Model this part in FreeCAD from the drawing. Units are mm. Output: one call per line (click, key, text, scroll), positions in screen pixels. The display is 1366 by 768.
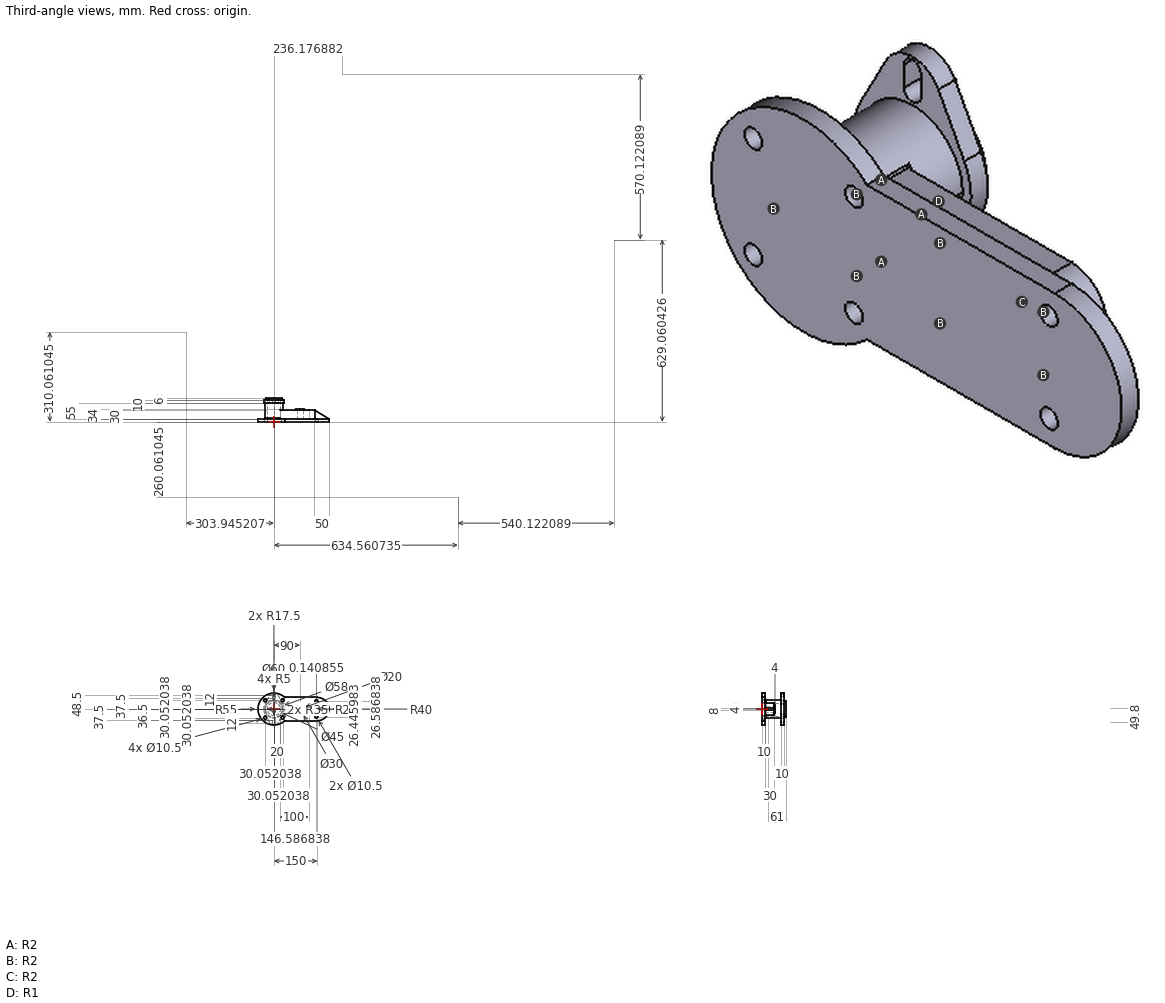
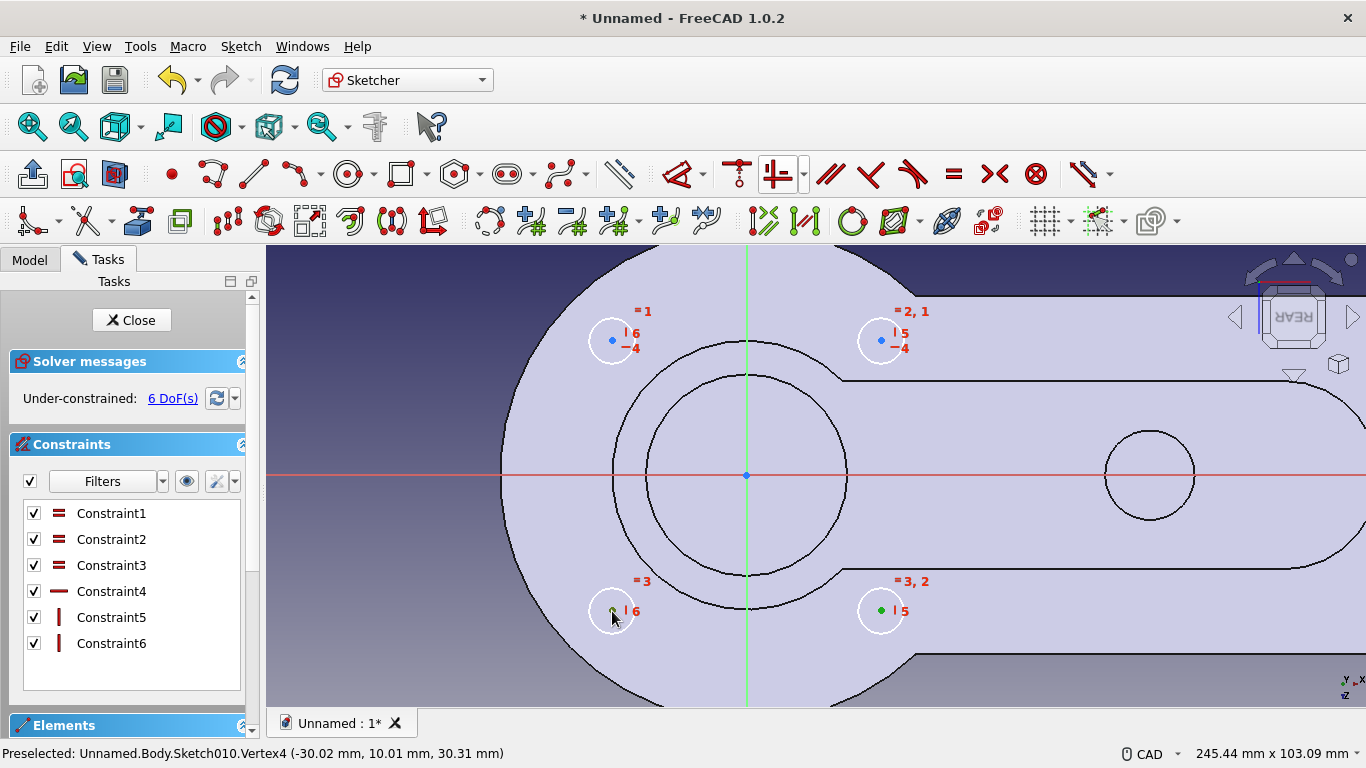
key(h)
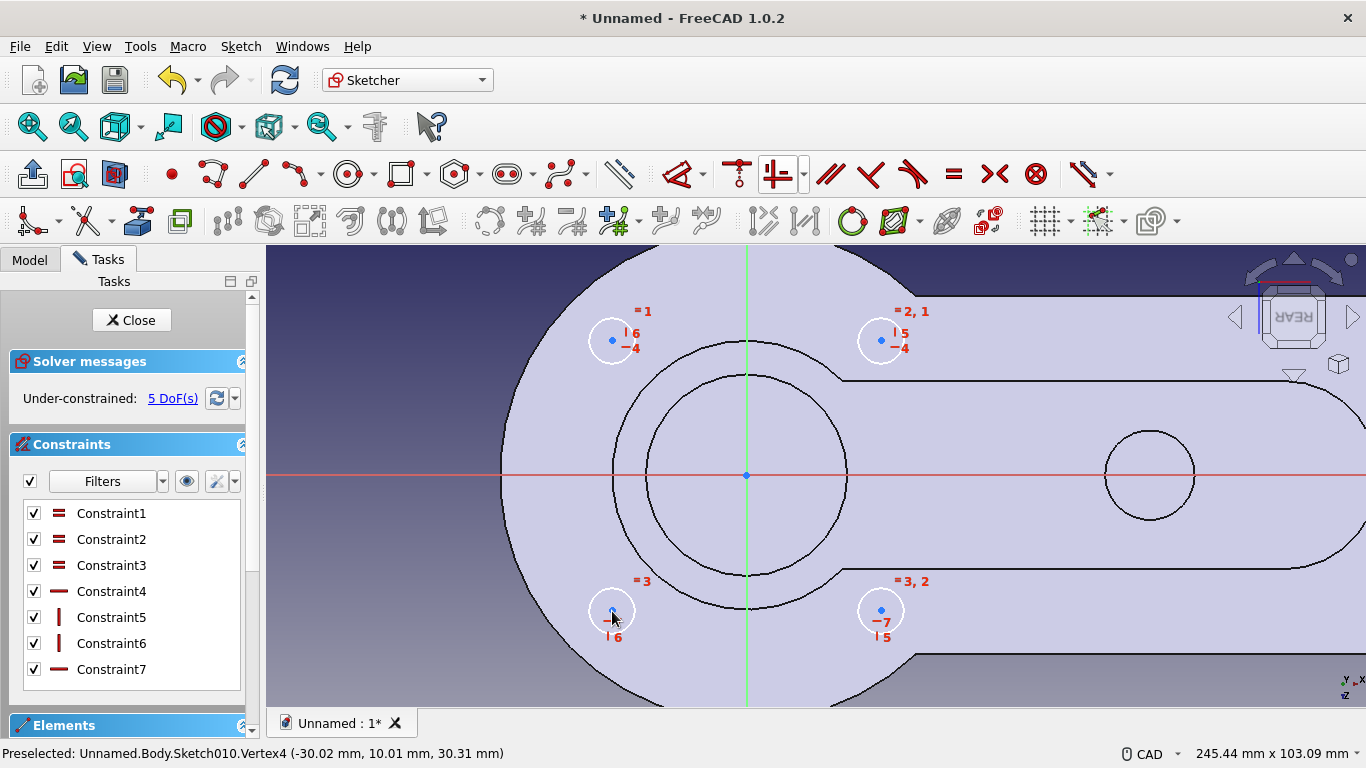
key(d)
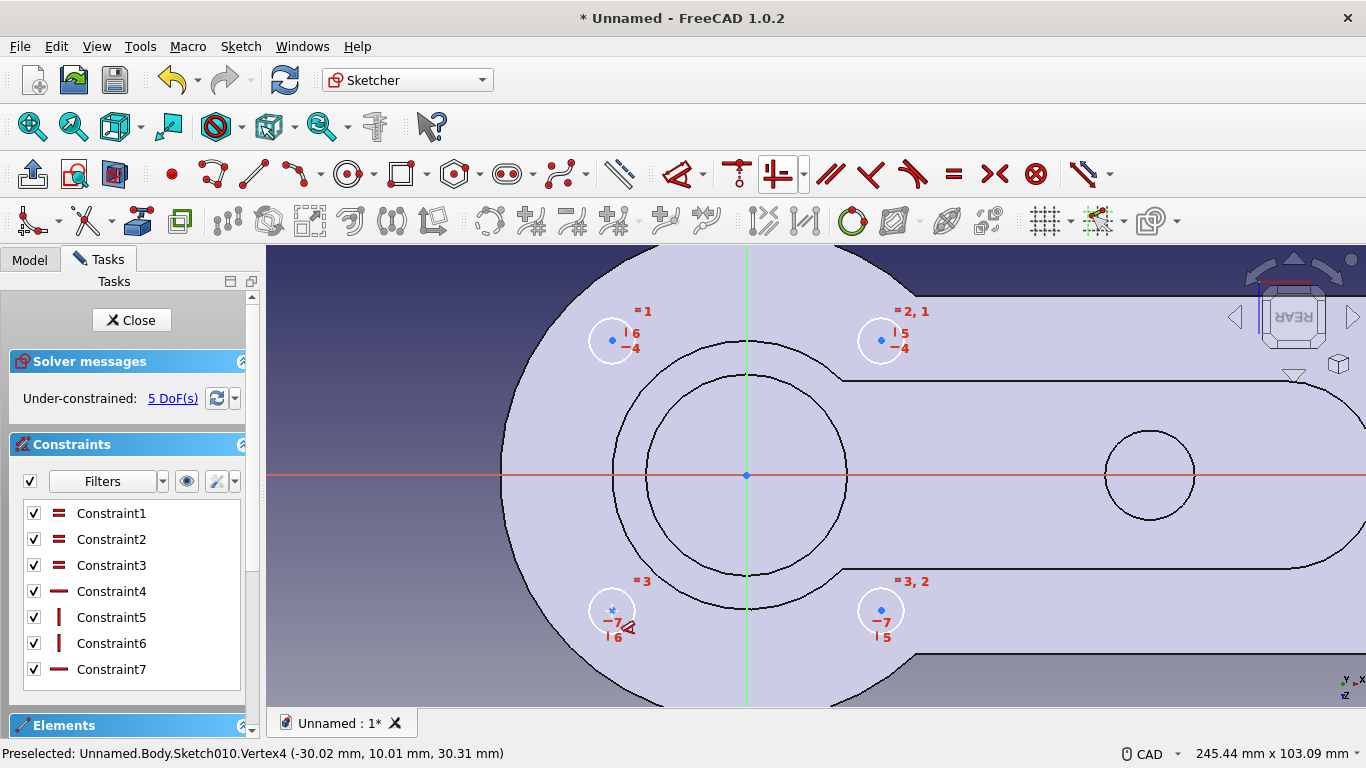
click(628, 325)
click(651, 302)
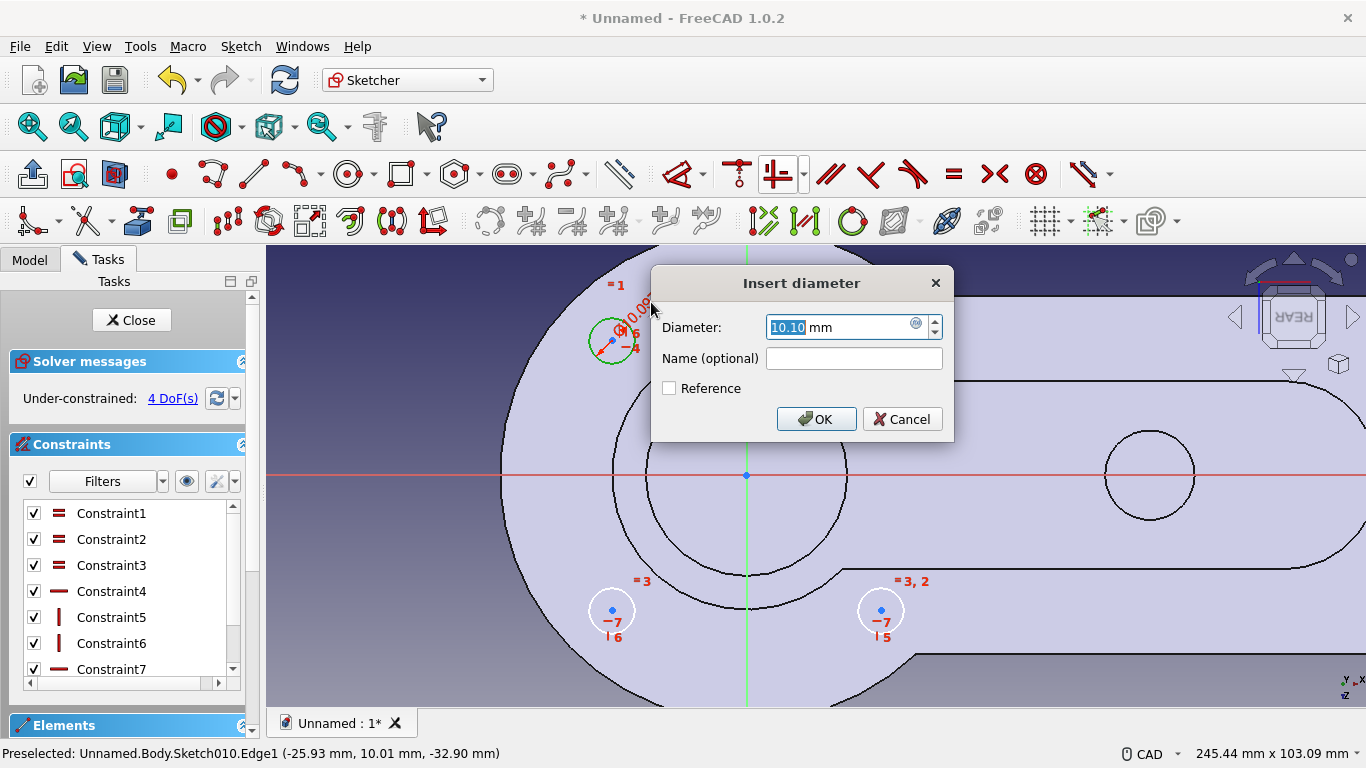
text(10.5)
key(Return)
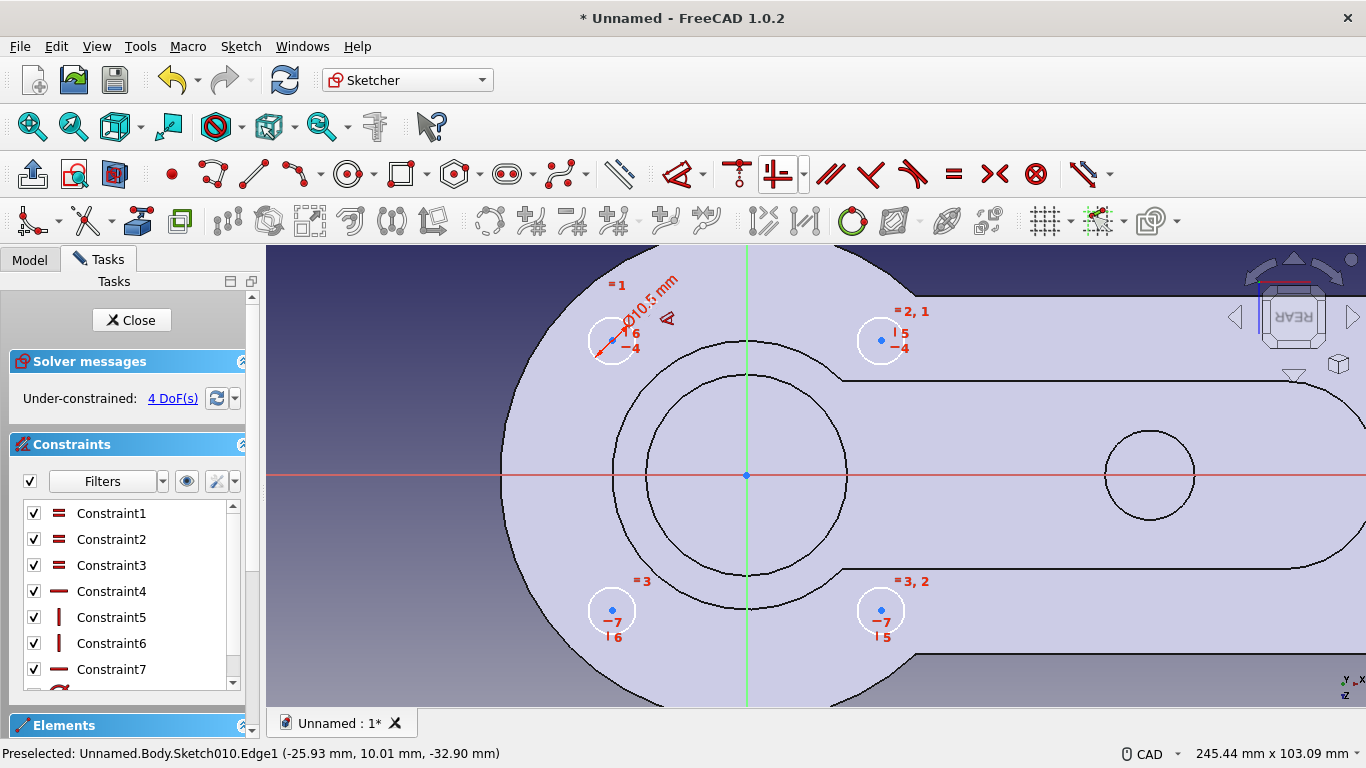
click(612, 341)
click(726, 307)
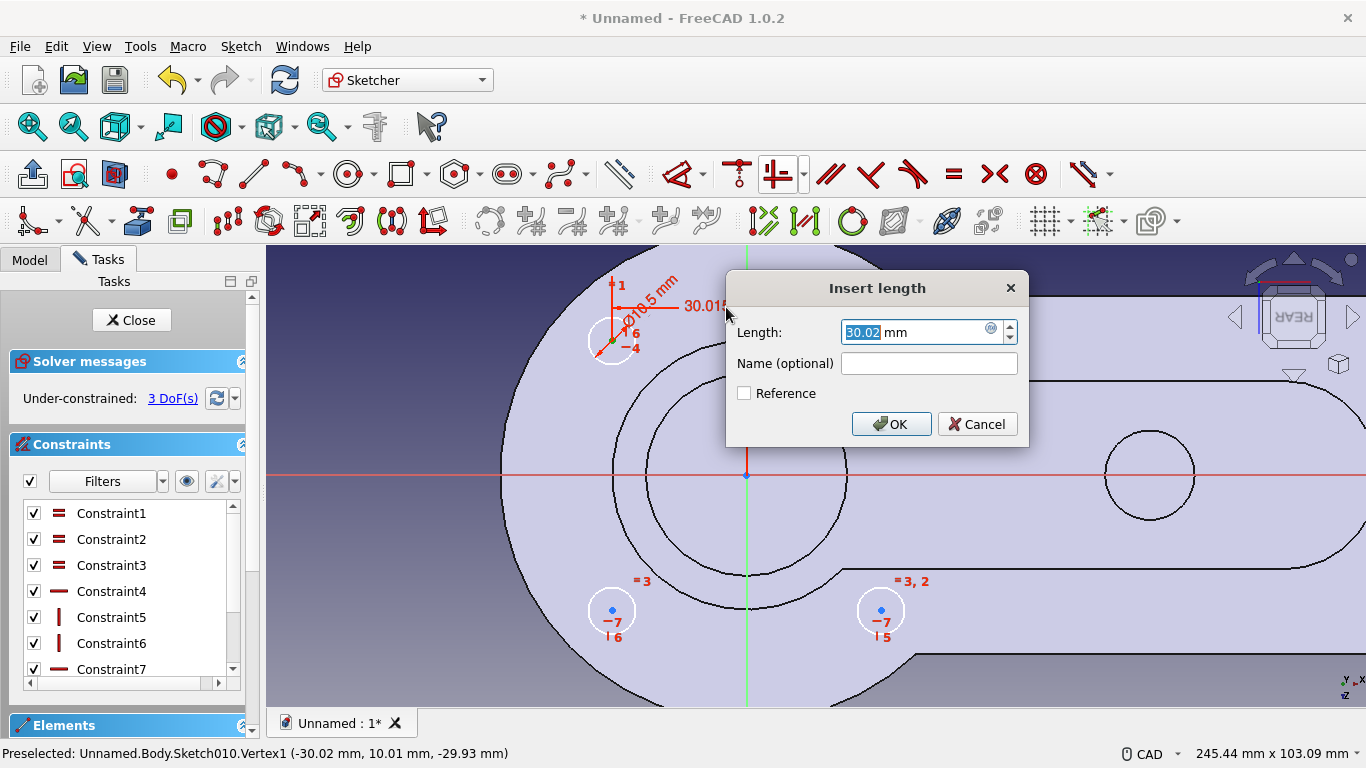
text(30.052038)
key(Return)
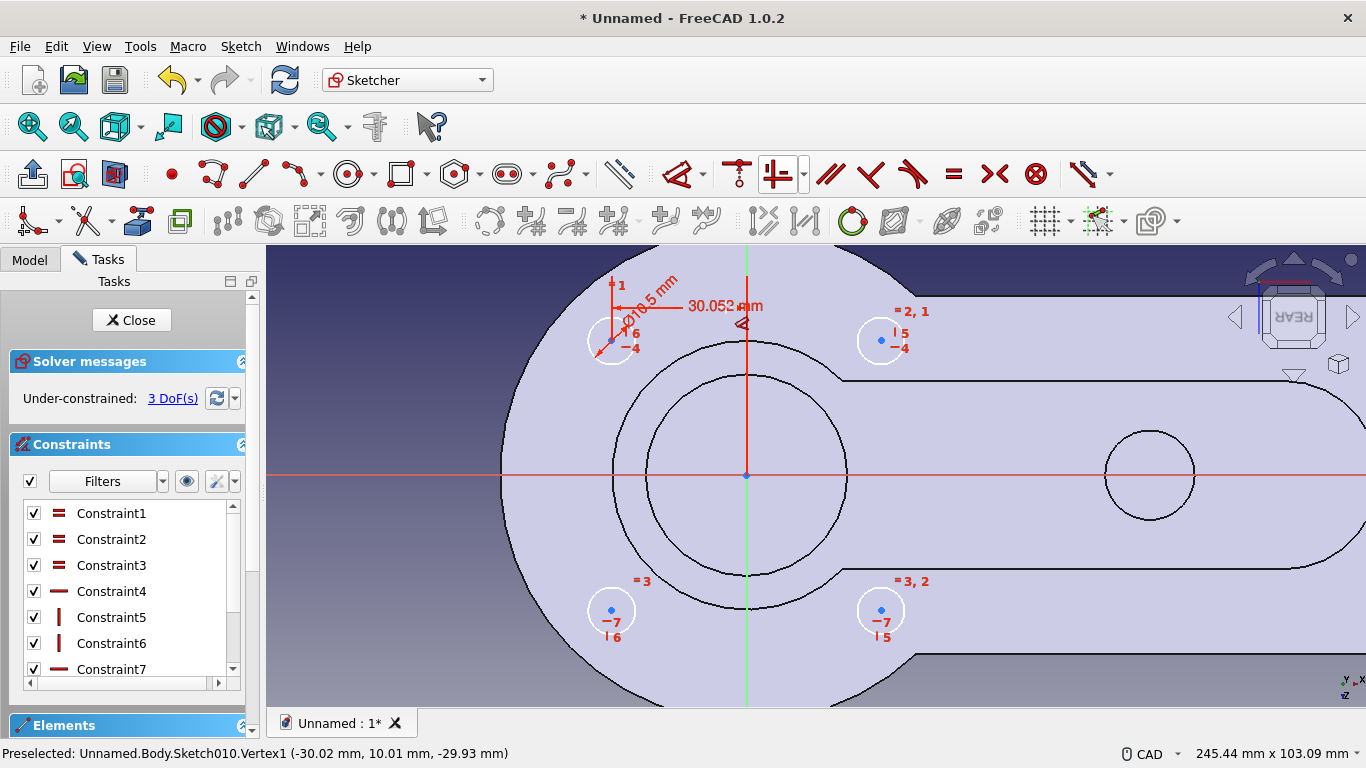
click(612, 341)
click(578, 408)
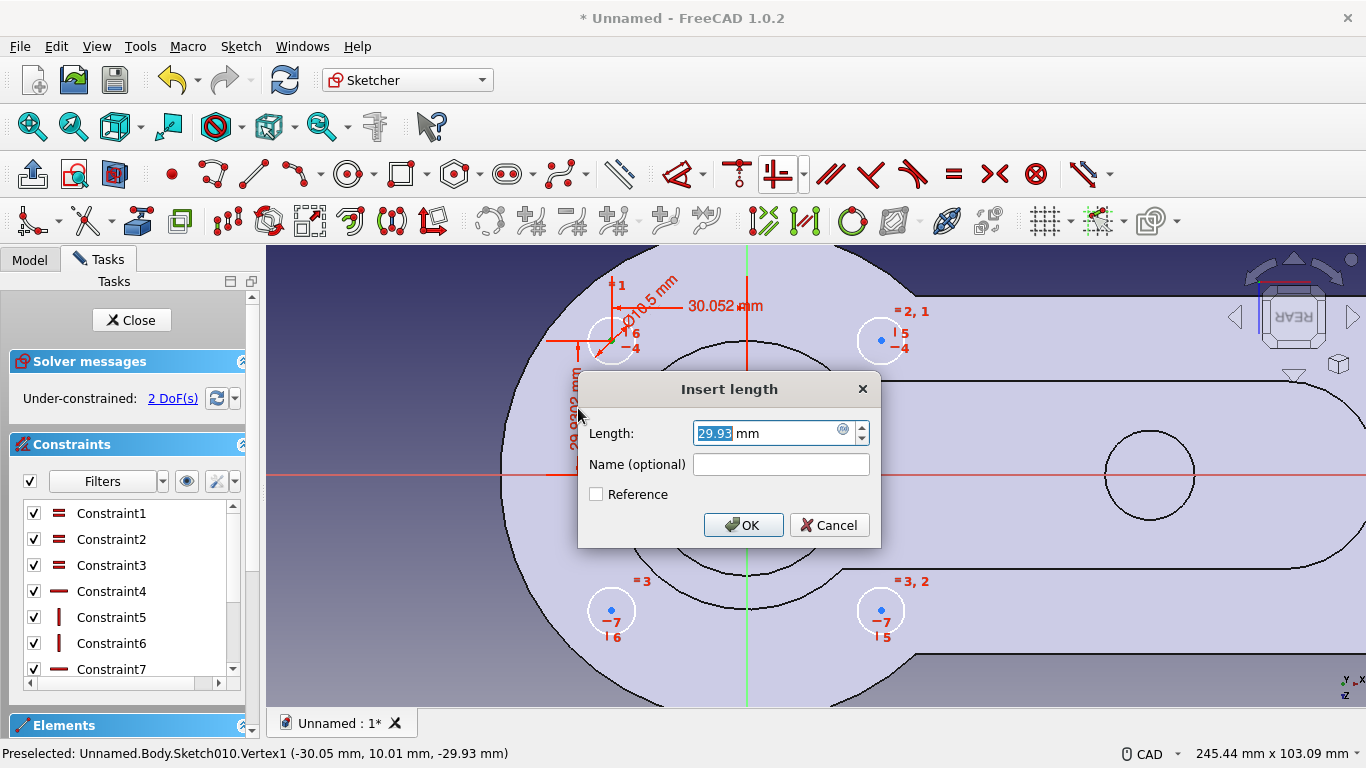
text(30.052038)
key(Return)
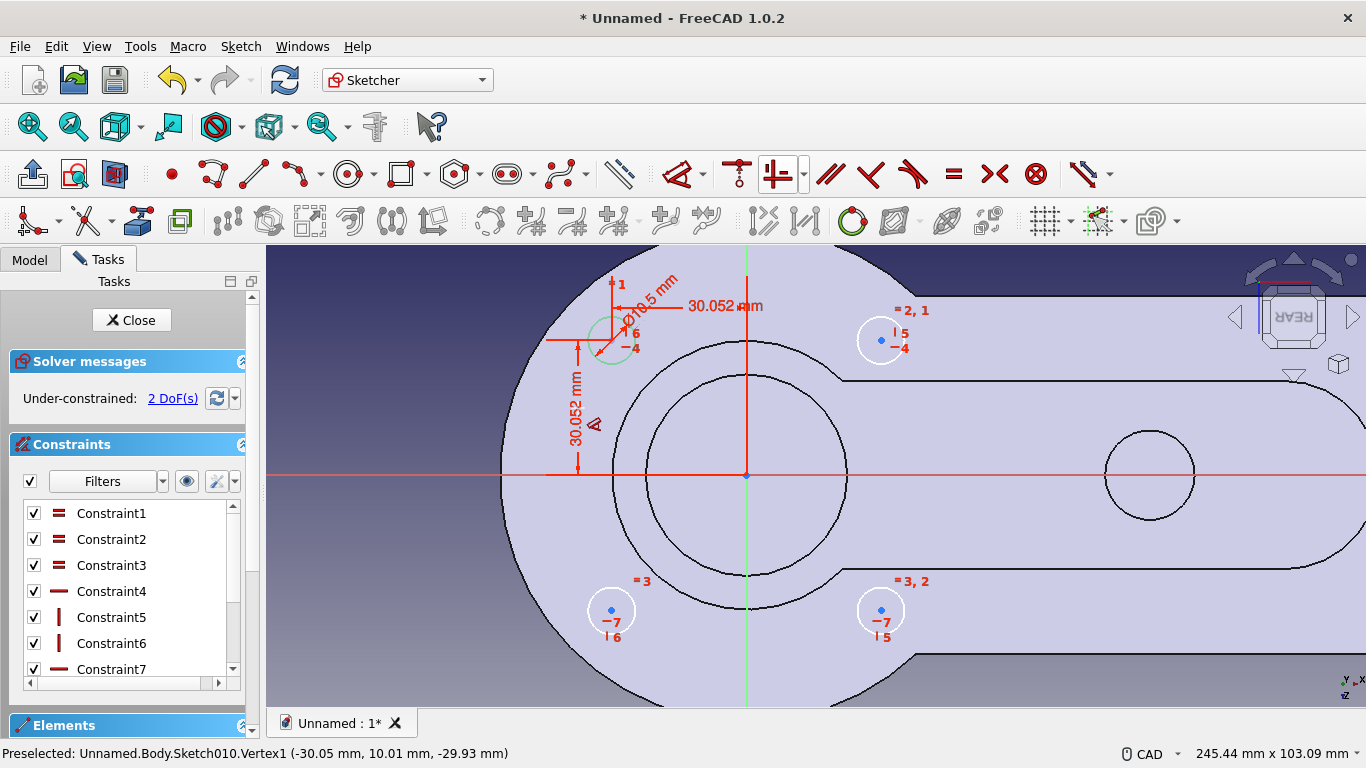
click(881, 340)
click(814, 306)